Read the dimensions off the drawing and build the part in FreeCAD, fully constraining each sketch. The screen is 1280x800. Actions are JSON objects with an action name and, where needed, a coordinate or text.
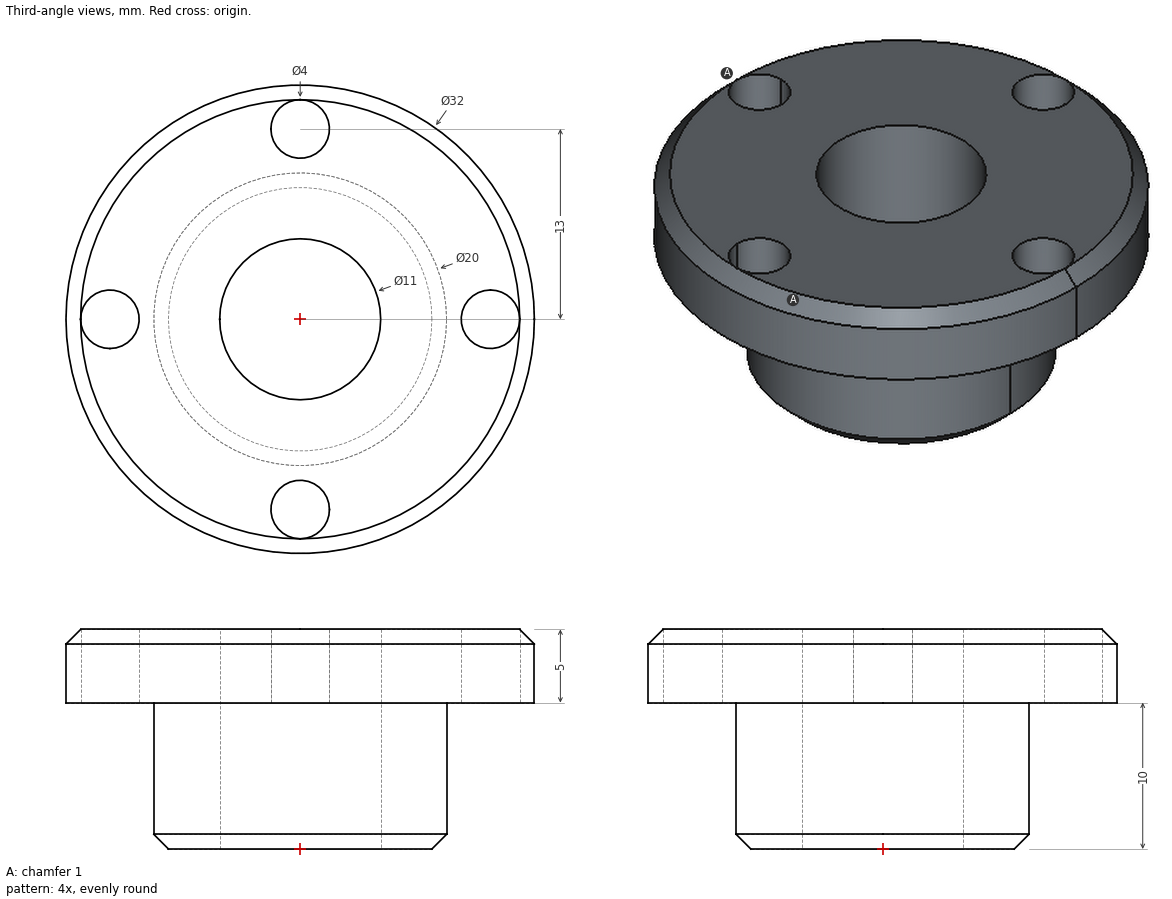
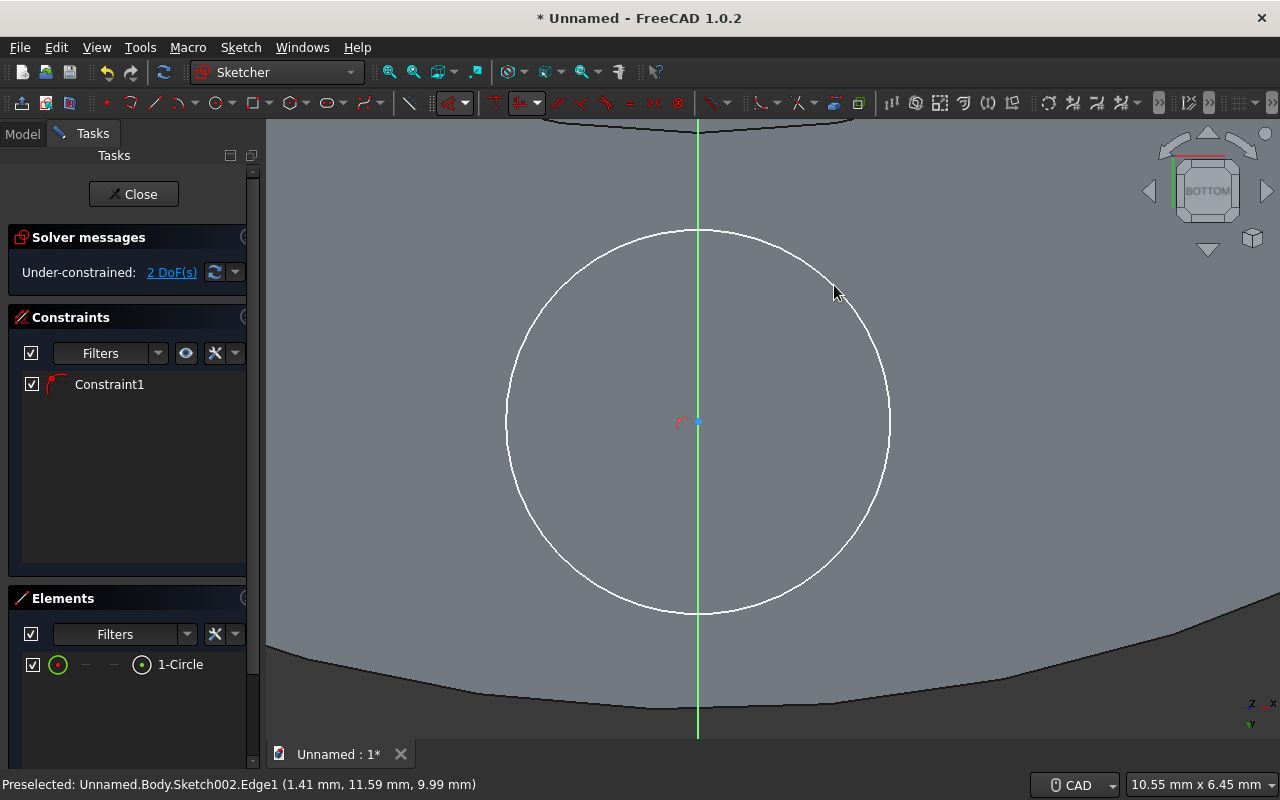
{"action": "left_click", "coordinate": [834, 286]}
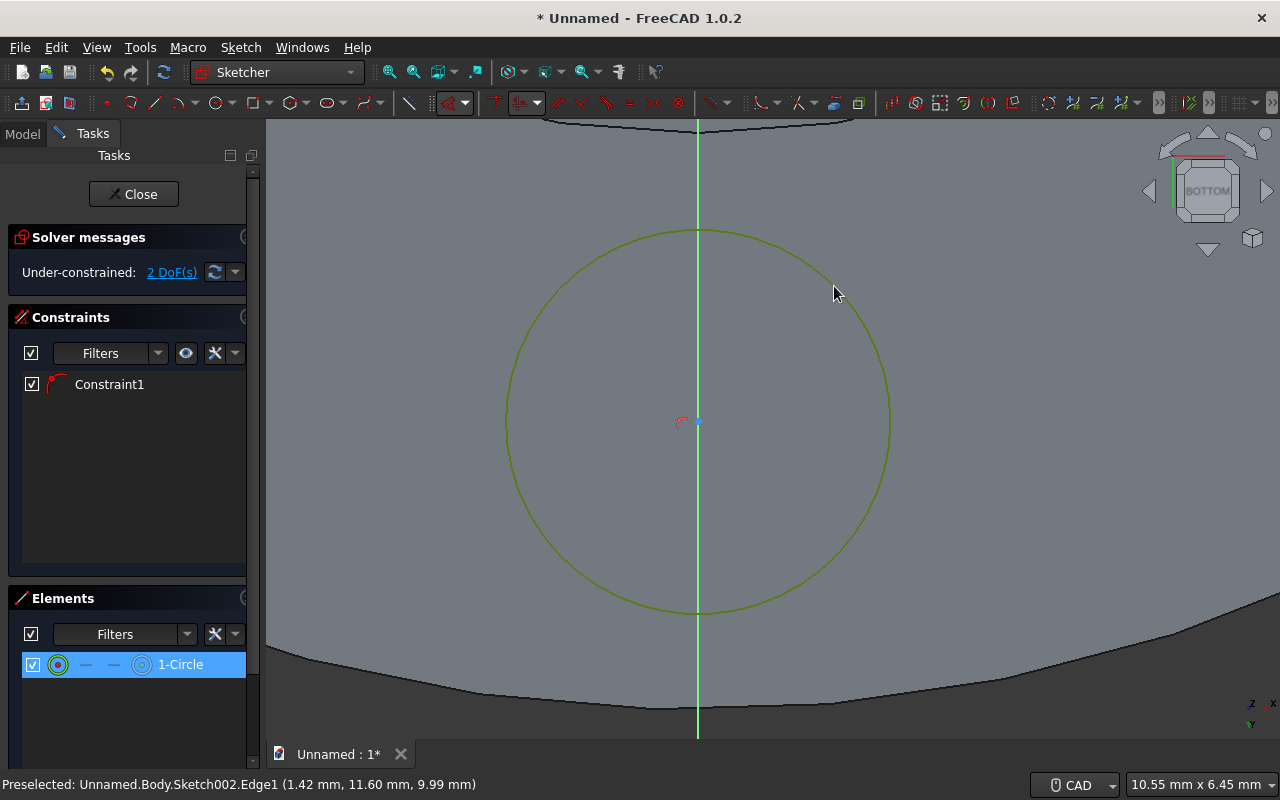
{"action": "left_click", "coordinate": [468, 104]}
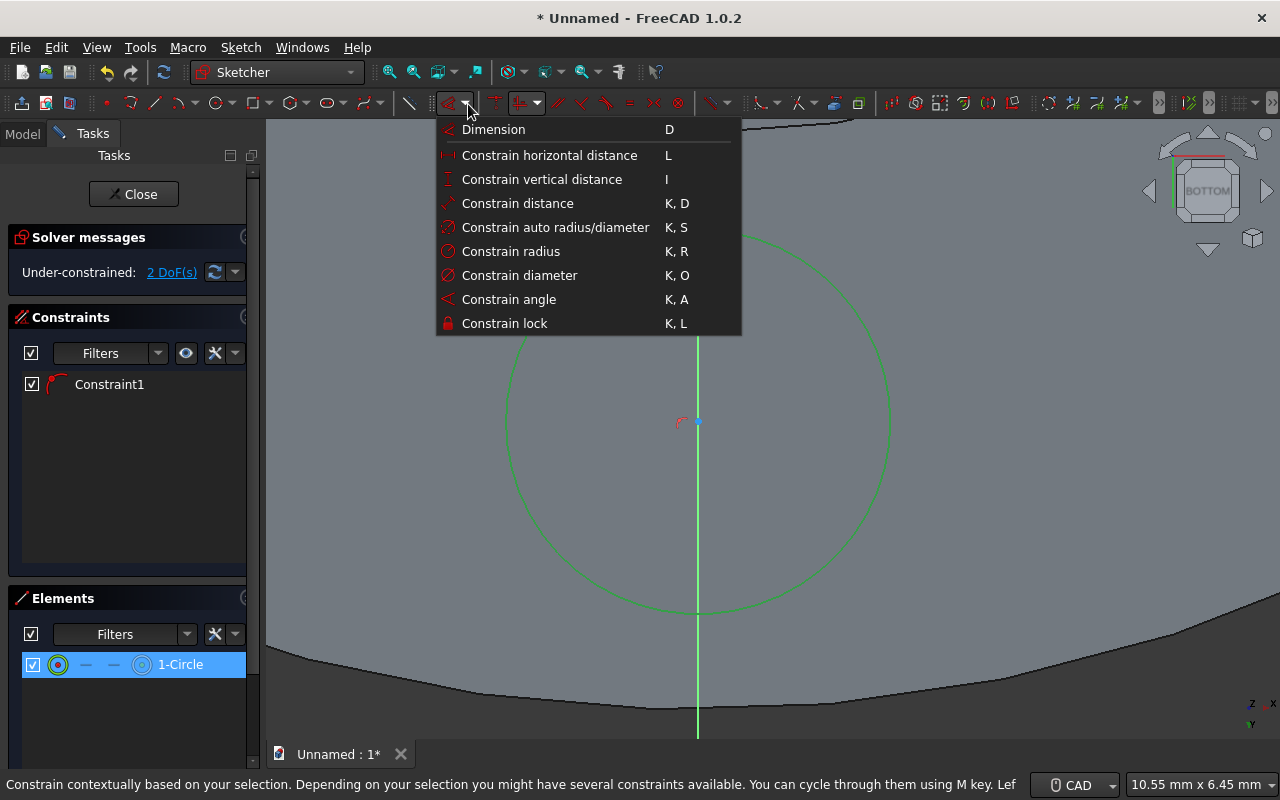
{"action": "left_click", "coordinate": [589, 275]}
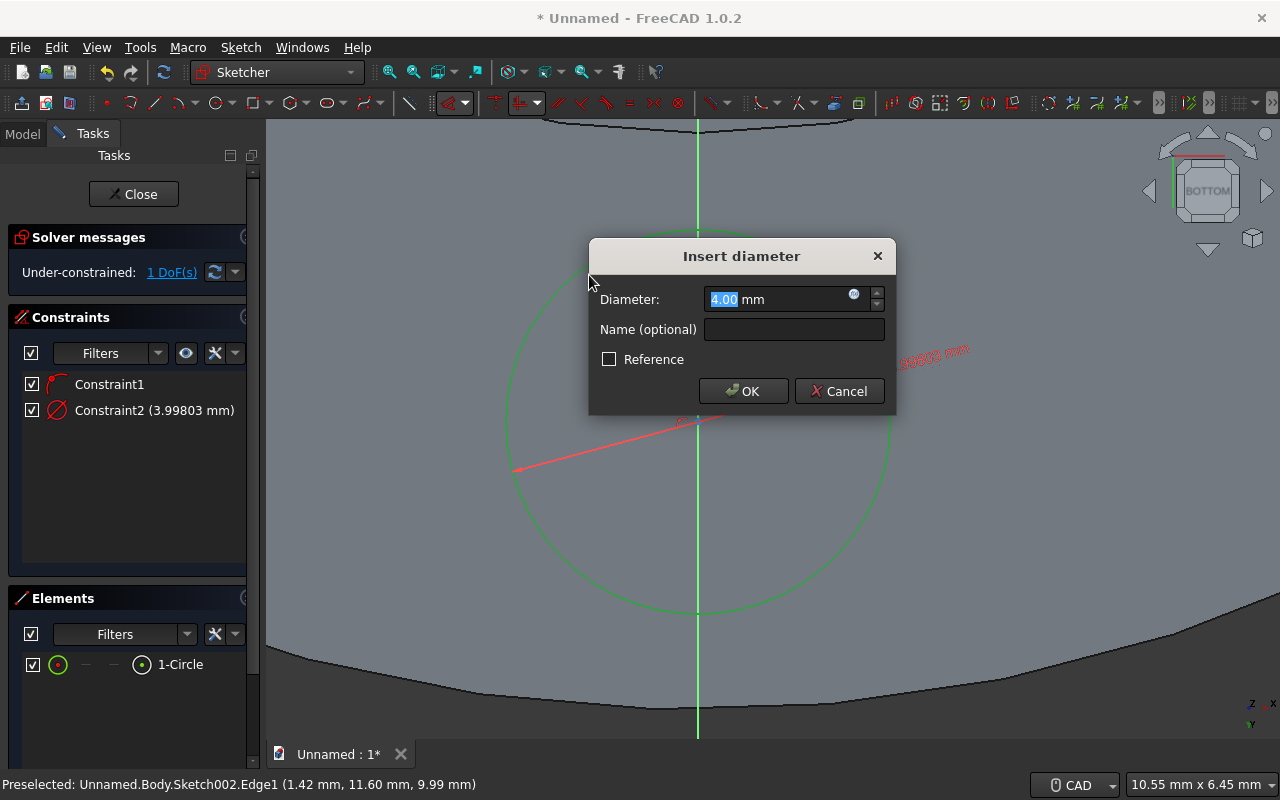
{"action": "type", "text": "4"}
{"action": "key", "text": "Return"}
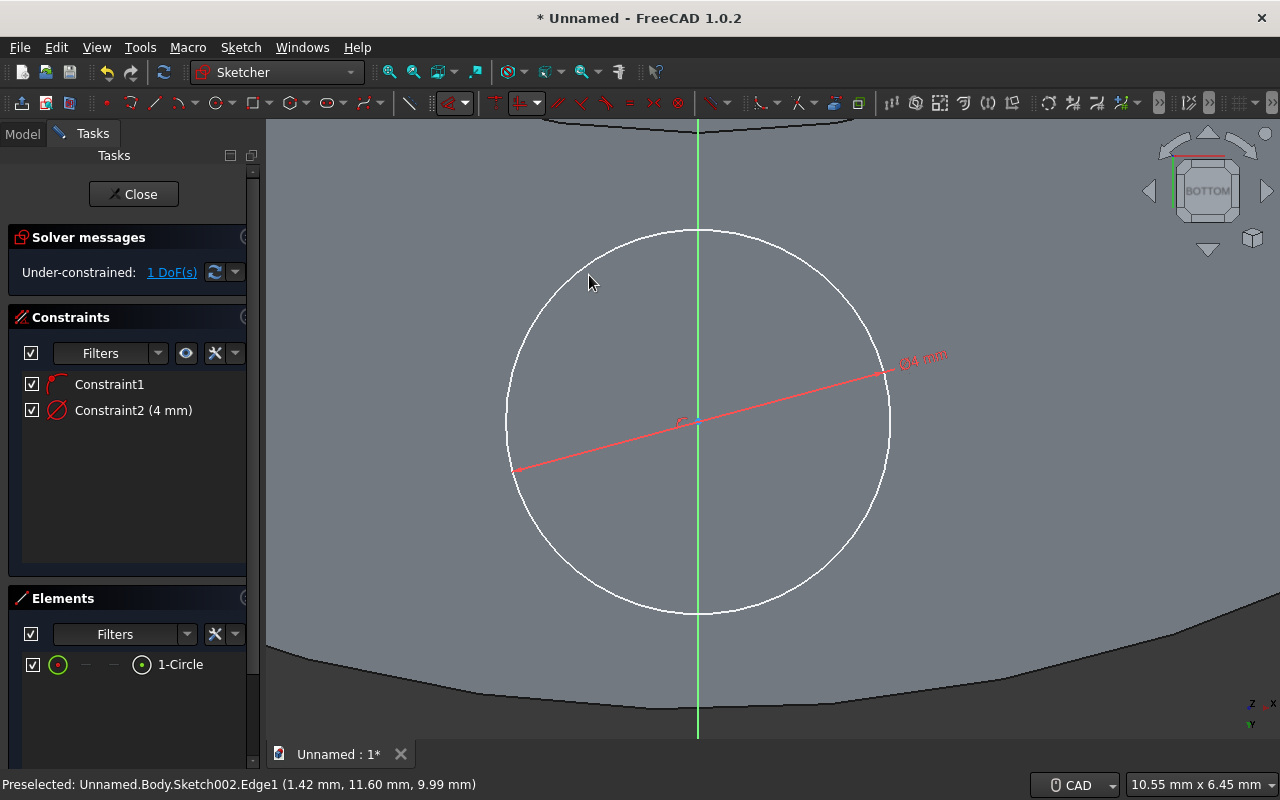
{"action": "left_click", "coordinate": [698, 422]}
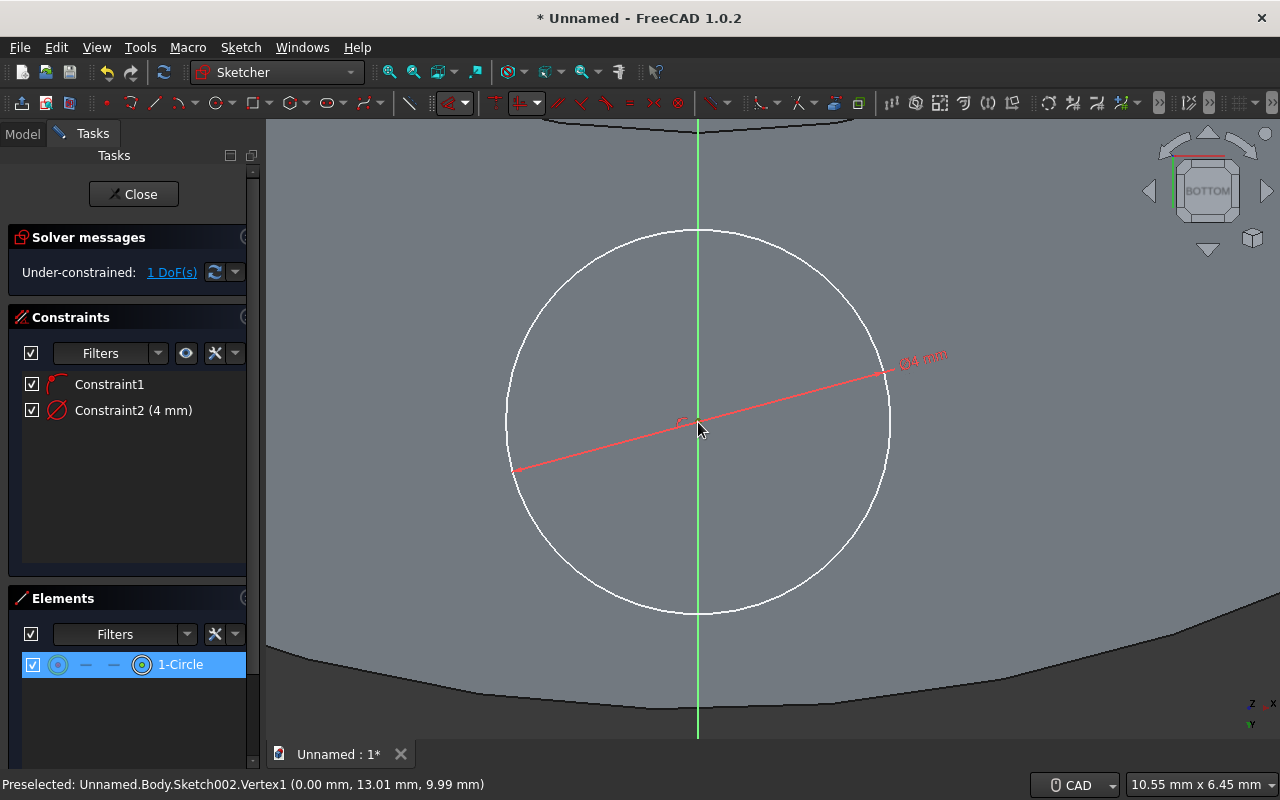
{"action": "left_click", "coordinate": [468, 104]}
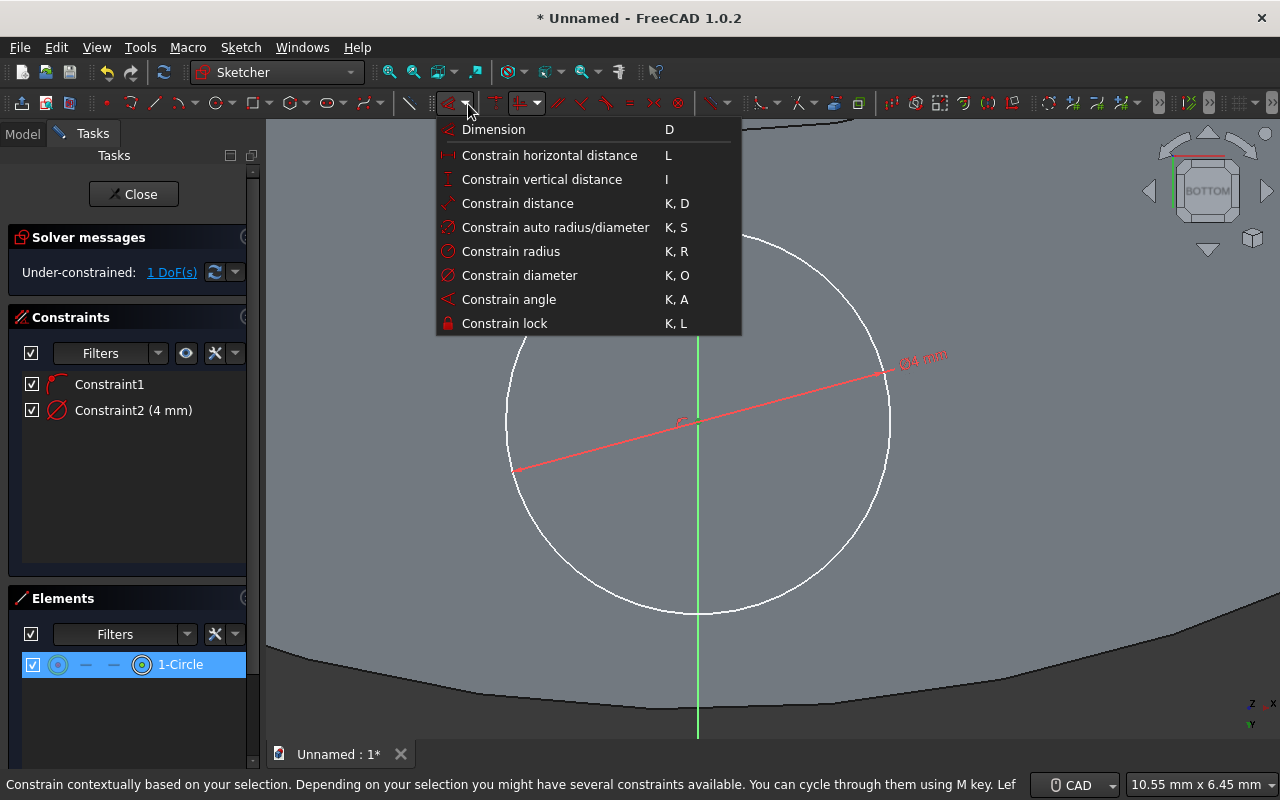
{"action": "left_click", "coordinate": [589, 179]}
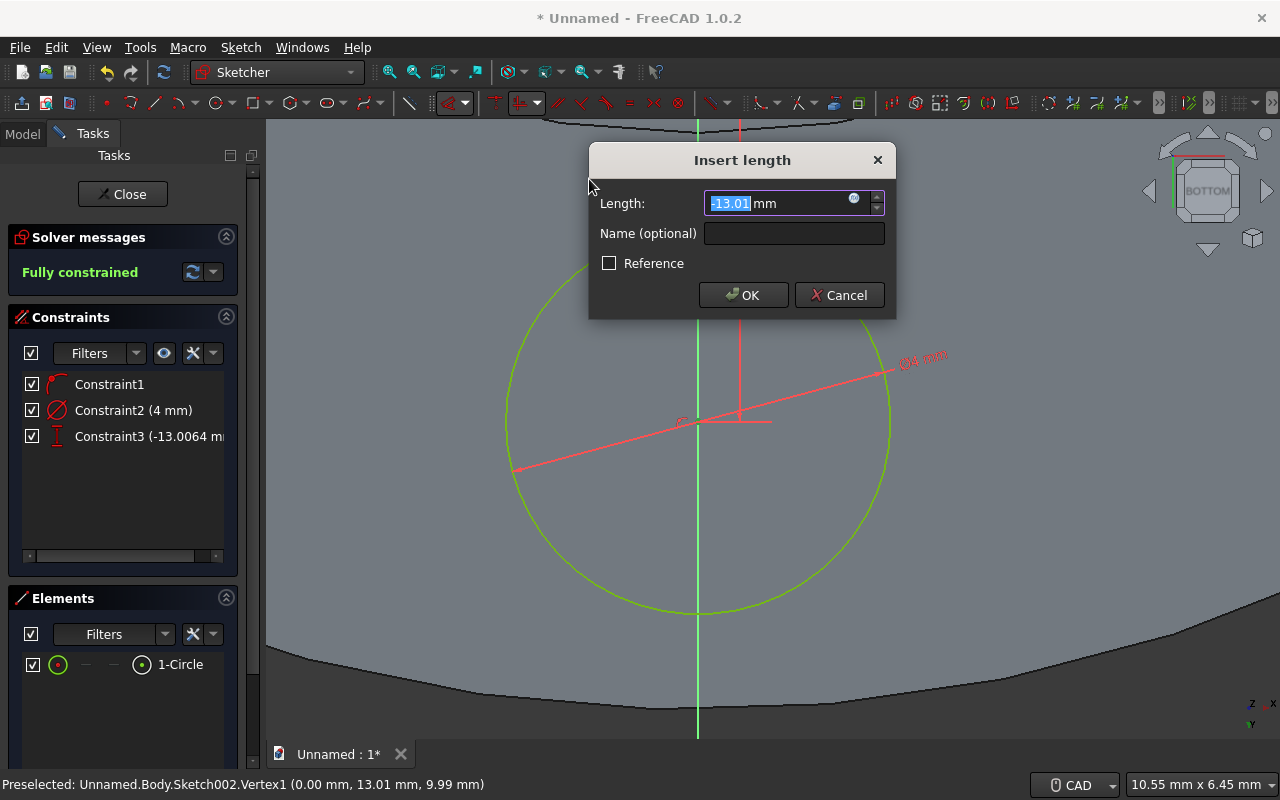
{"action": "type", "text": "-13"}
{"action": "key", "text": "Return"}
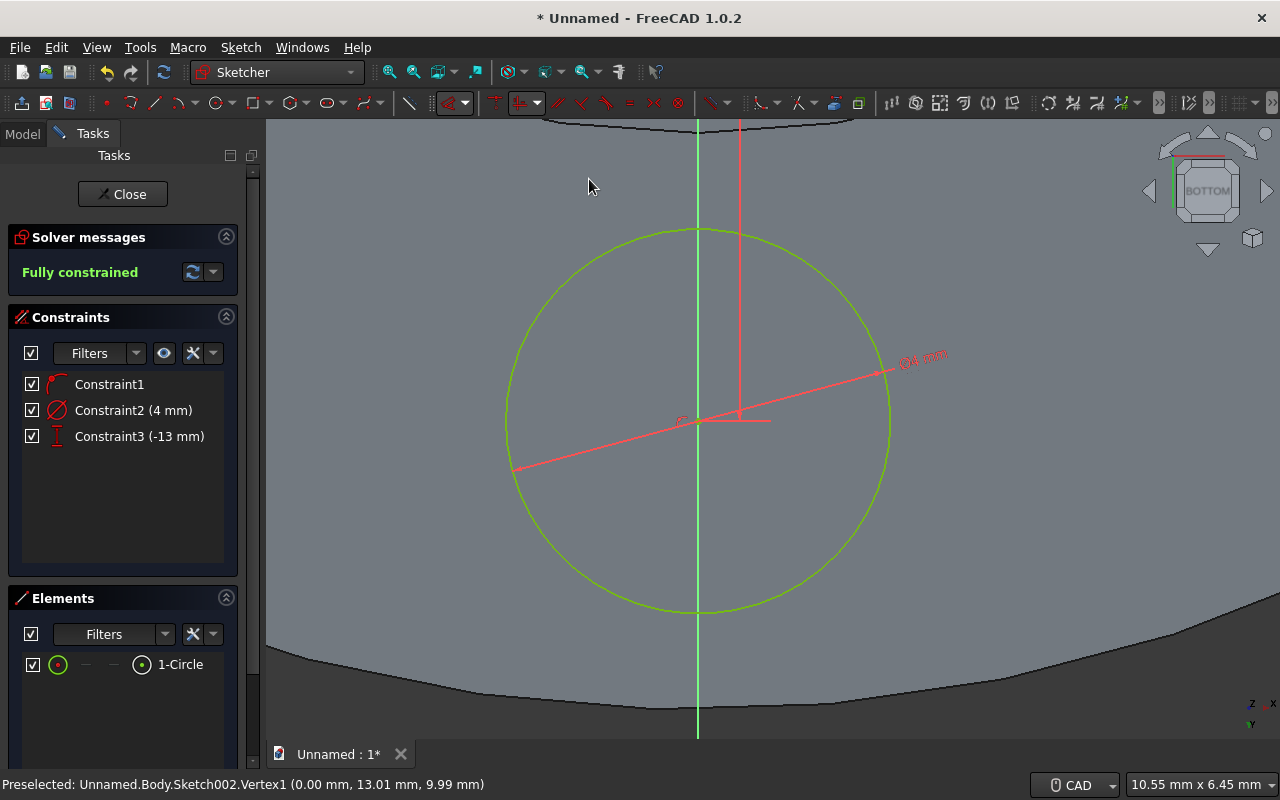
{"action": "left_click", "coordinate": [123, 194]}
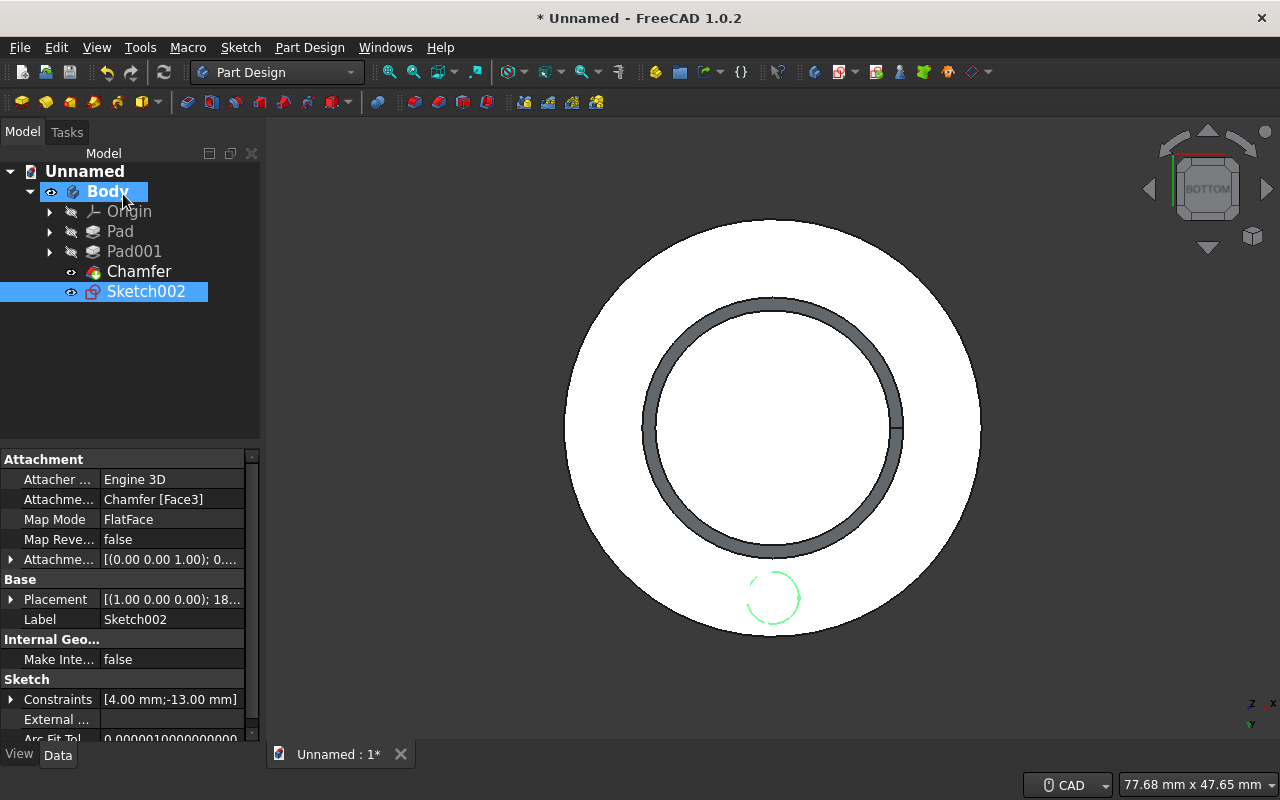
{"action": "left_click", "coordinate": [188, 102]}